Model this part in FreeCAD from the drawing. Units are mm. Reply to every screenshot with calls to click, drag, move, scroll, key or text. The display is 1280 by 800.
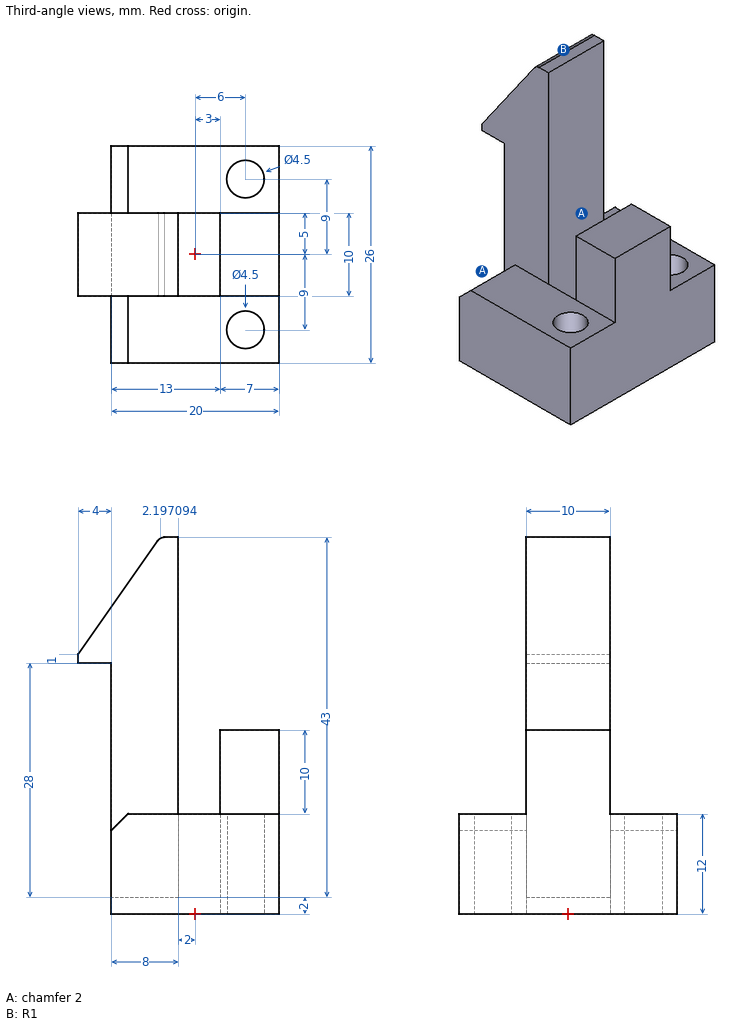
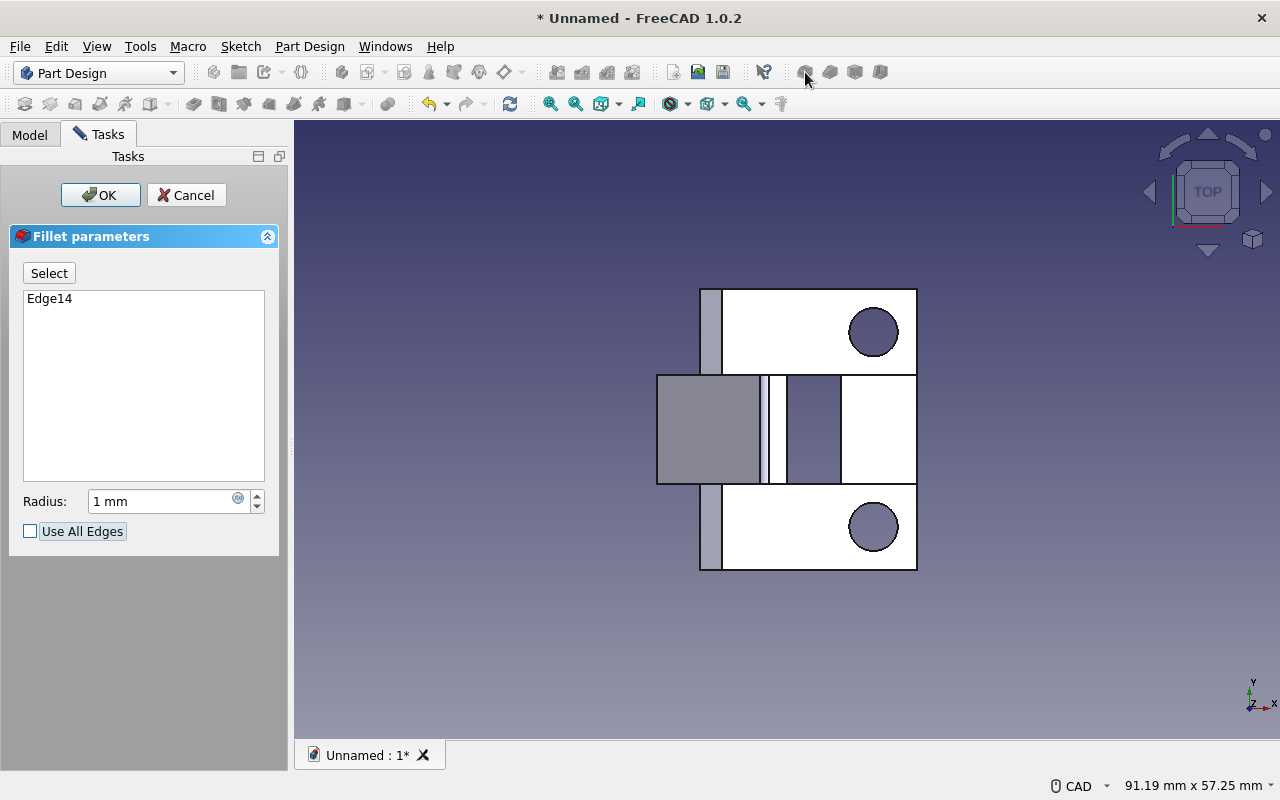
click(101, 195)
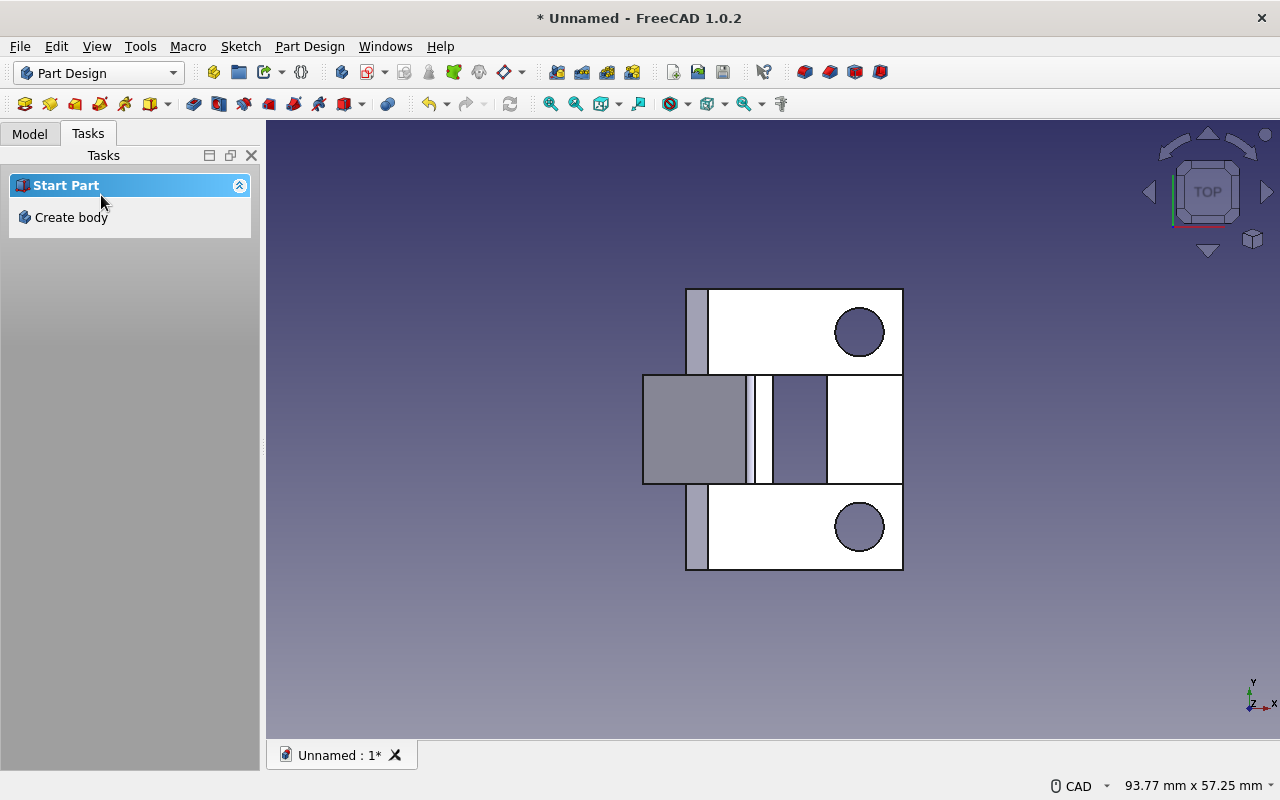
key(0)